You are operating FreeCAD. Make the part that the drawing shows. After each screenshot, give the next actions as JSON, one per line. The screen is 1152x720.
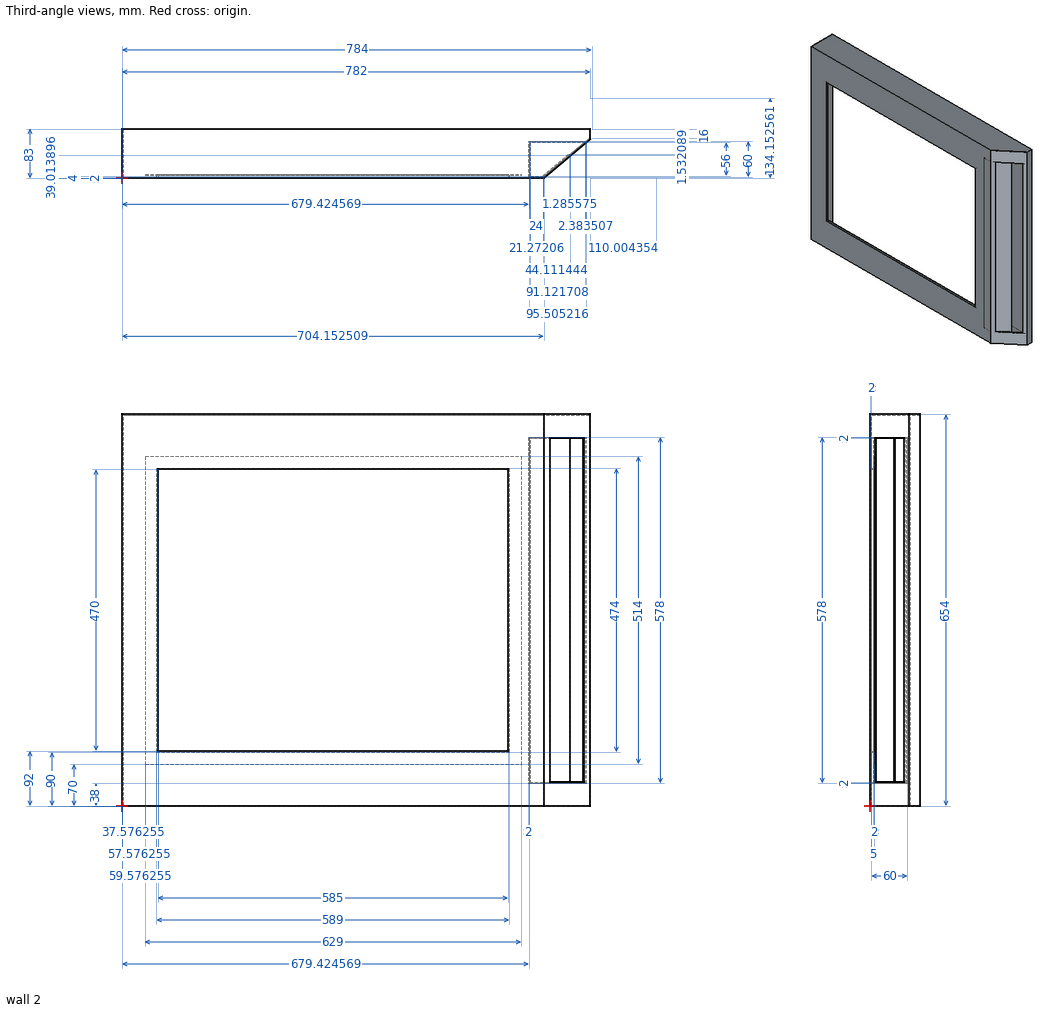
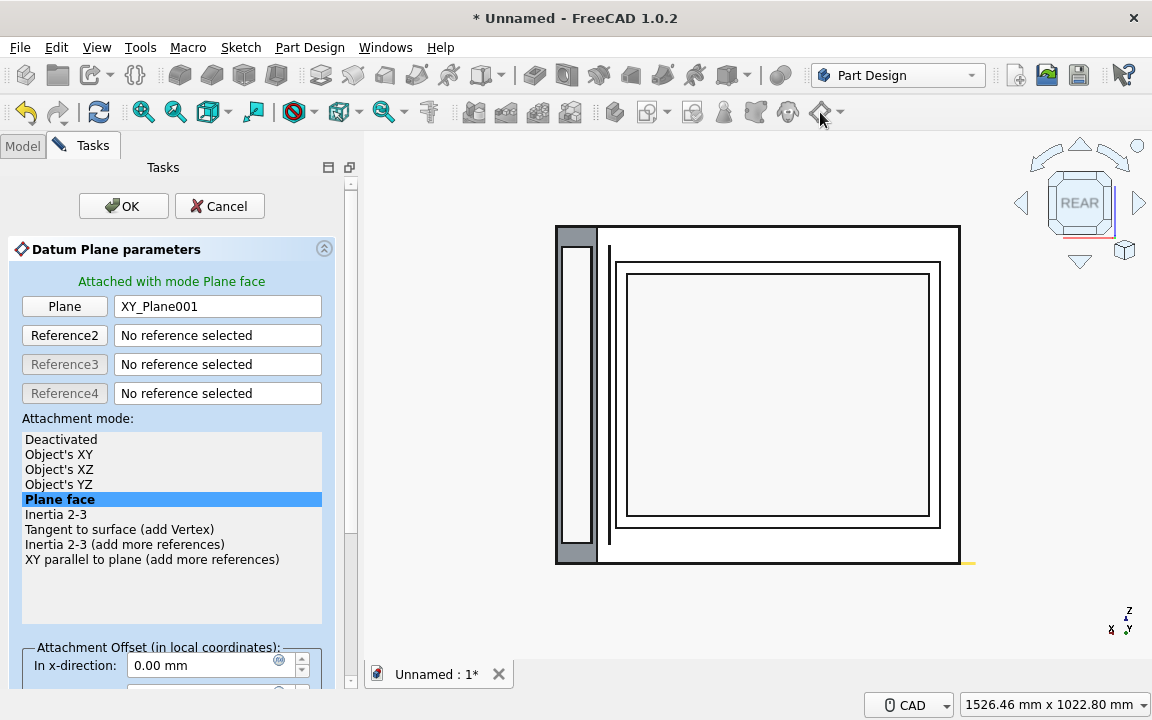
{"action": "scroll", "coordinate": [351, 432], "scroll_direction": "down", "scroll_amount": 2}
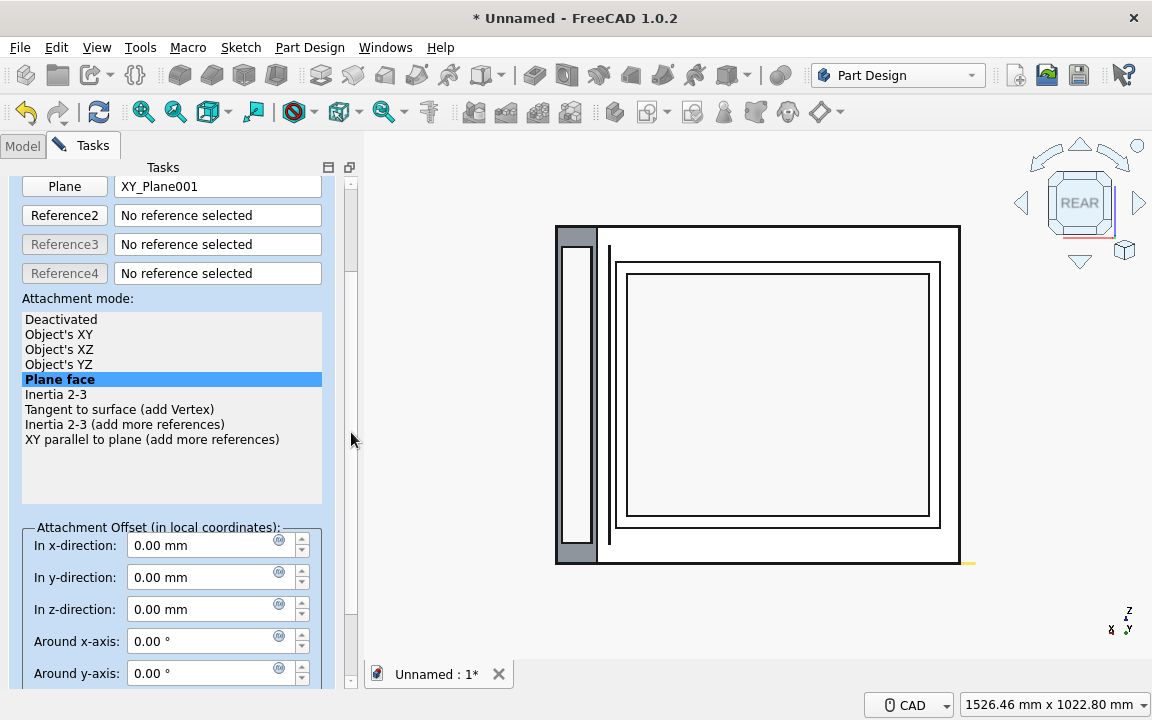
{"action": "triple_click", "coordinate": [210, 609]}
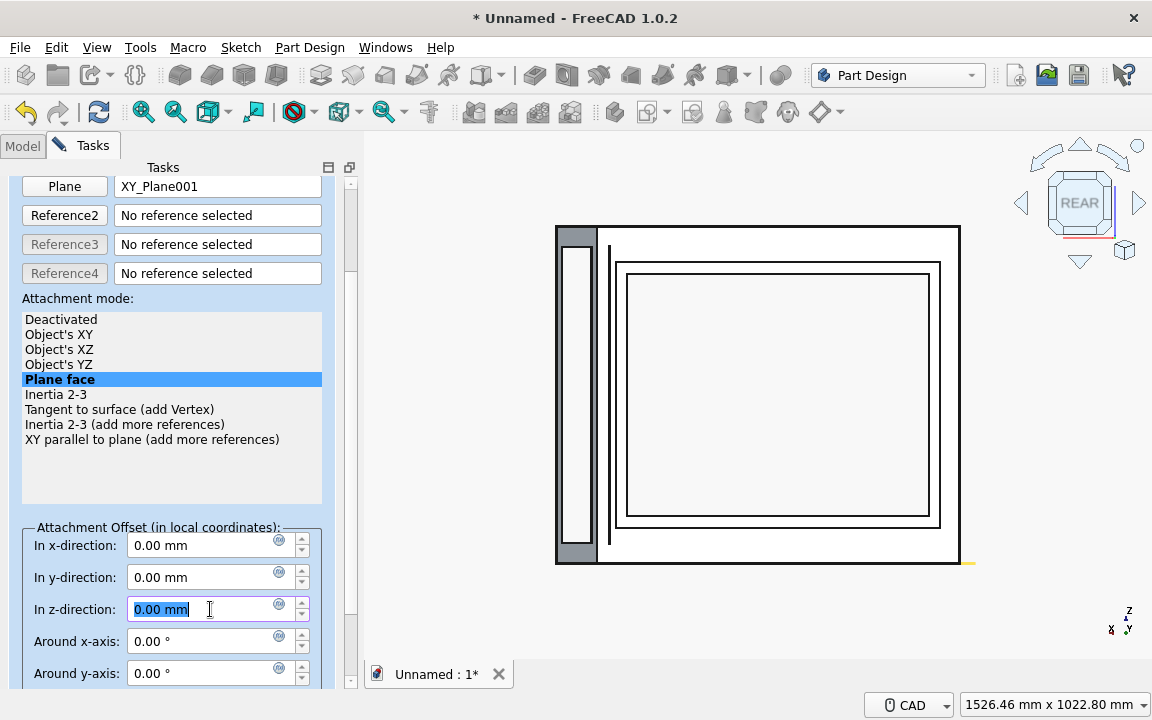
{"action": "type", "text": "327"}
{"action": "key", "text": "Tab"}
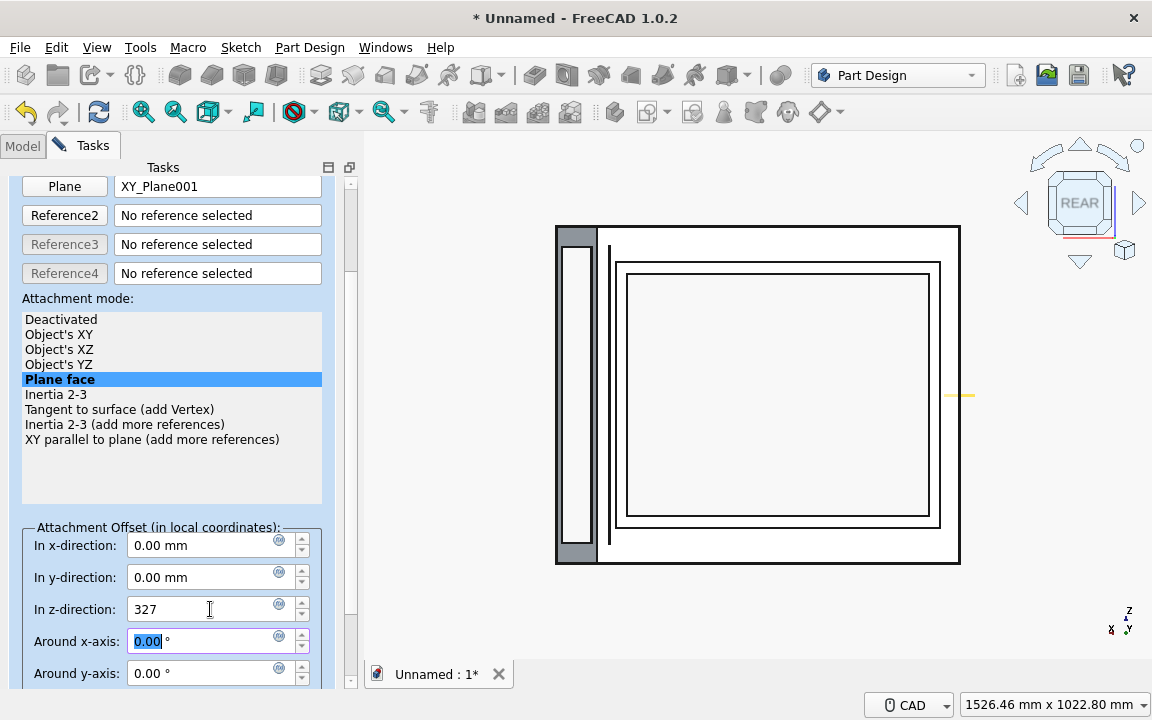
{"action": "scroll", "coordinate": [351, 432], "scroll_direction": "up", "scroll_amount": 3}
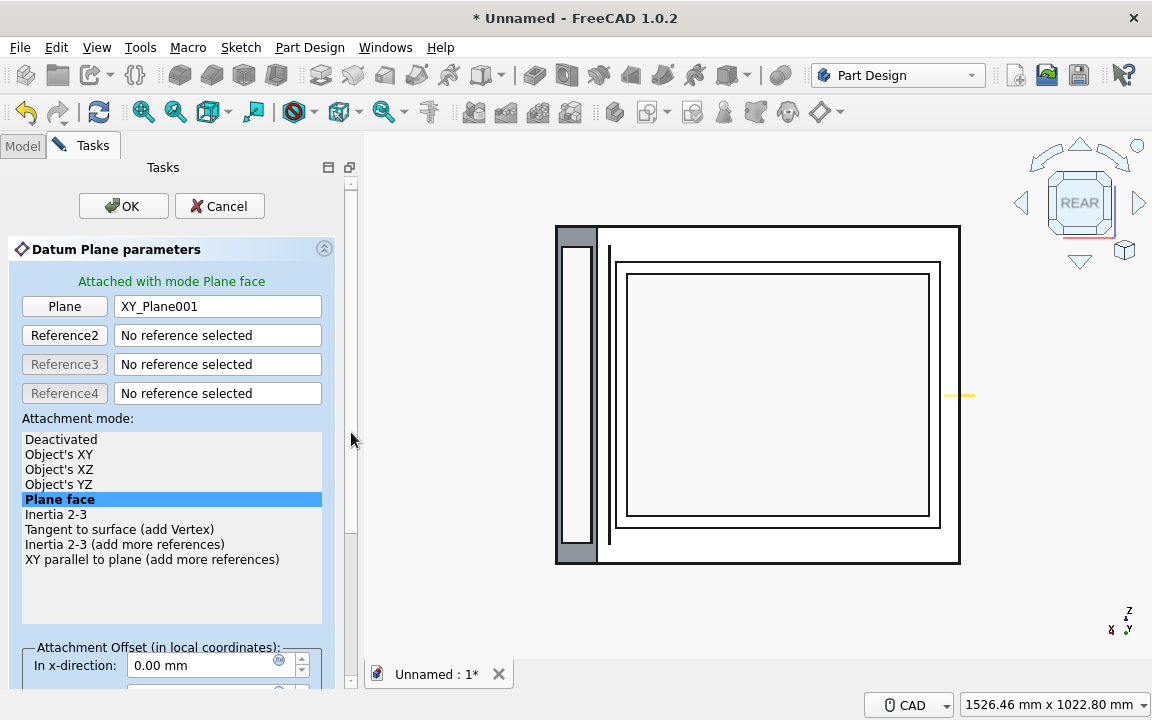
{"action": "left_click", "coordinate": [124, 206]}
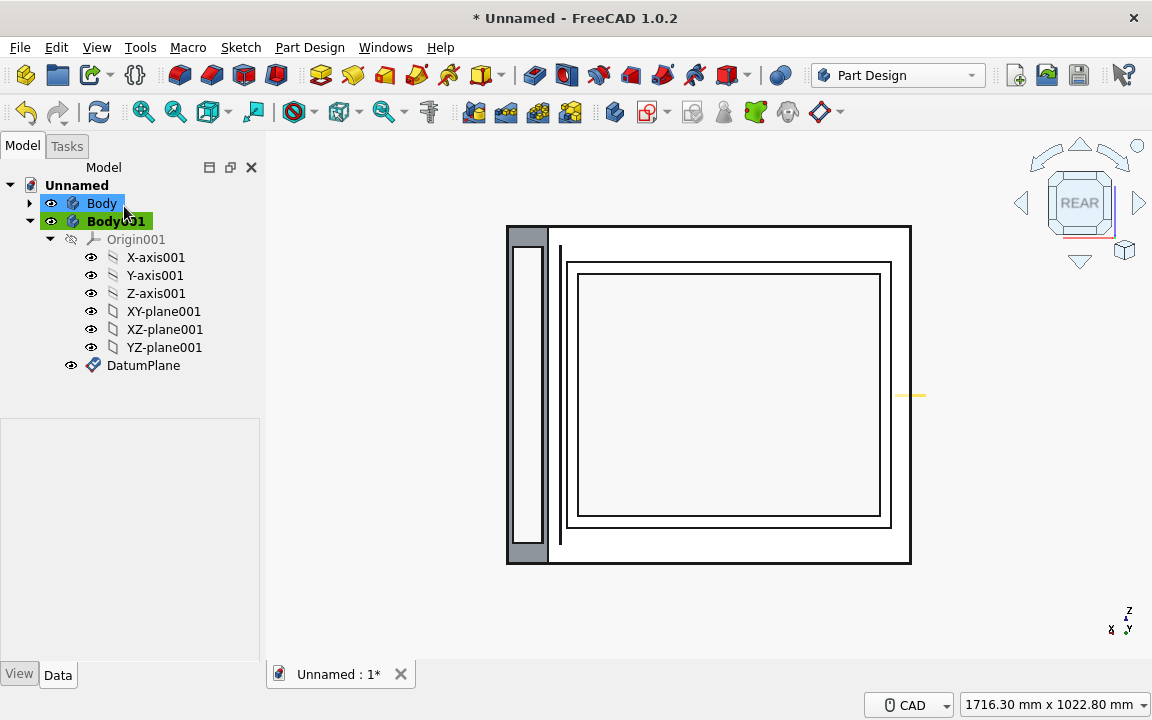
{"action": "left_click", "coordinate": [116, 365]}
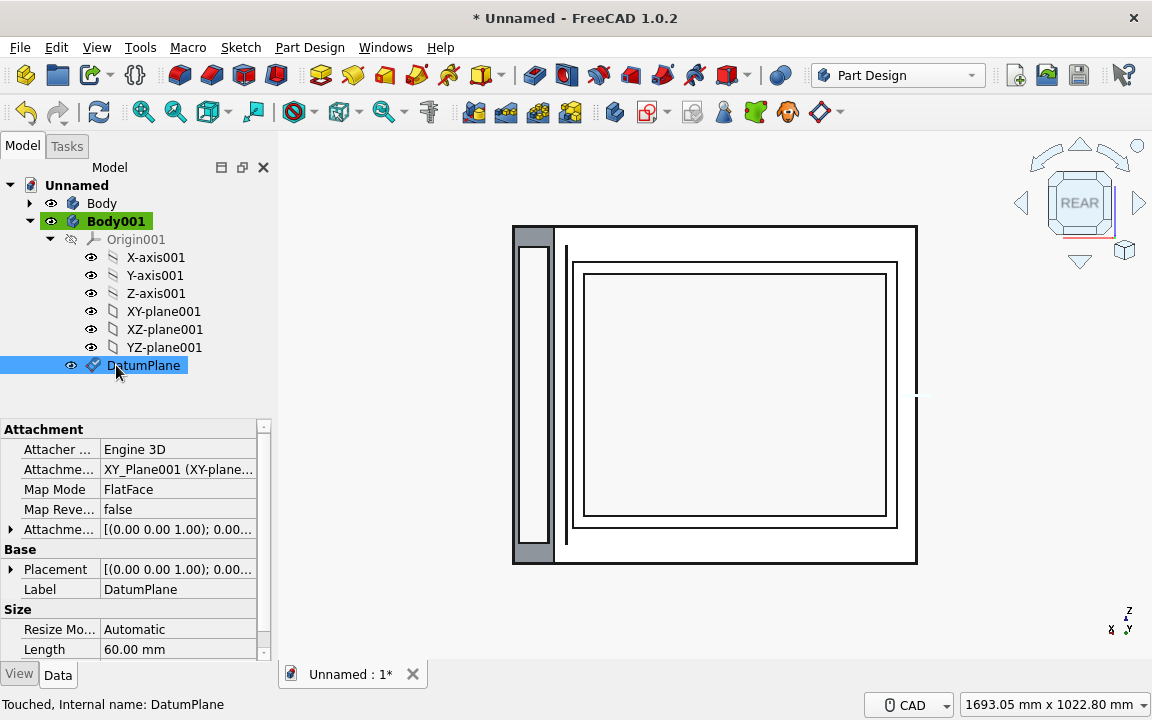
{"action": "left_click", "coordinate": [648, 112]}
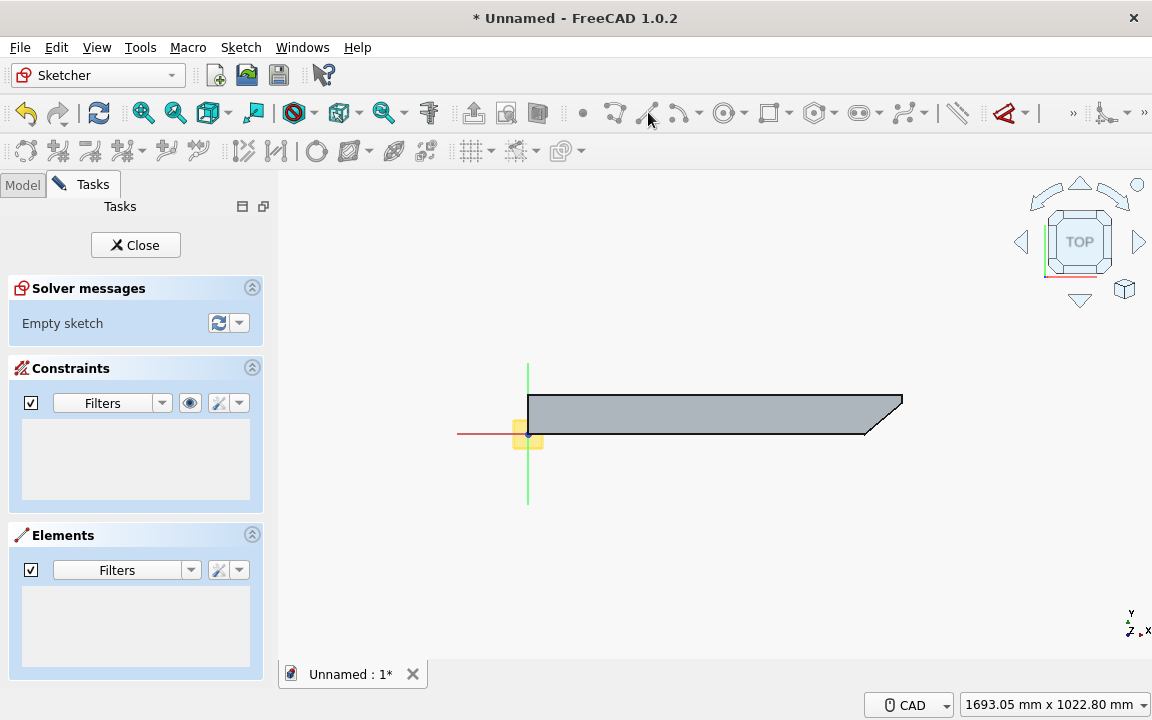
{"action": "scroll", "coordinate": [893, 419], "scroll_direction": "up", "scroll_amount": 12}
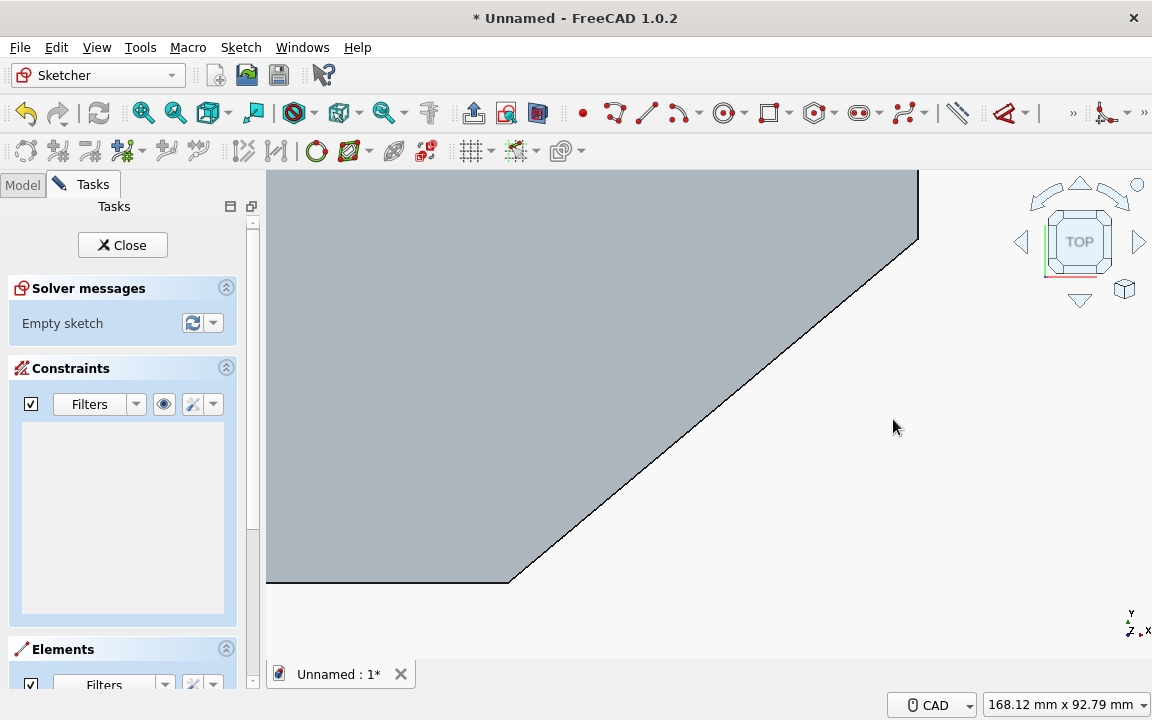
{"action": "key", "text": "g m"}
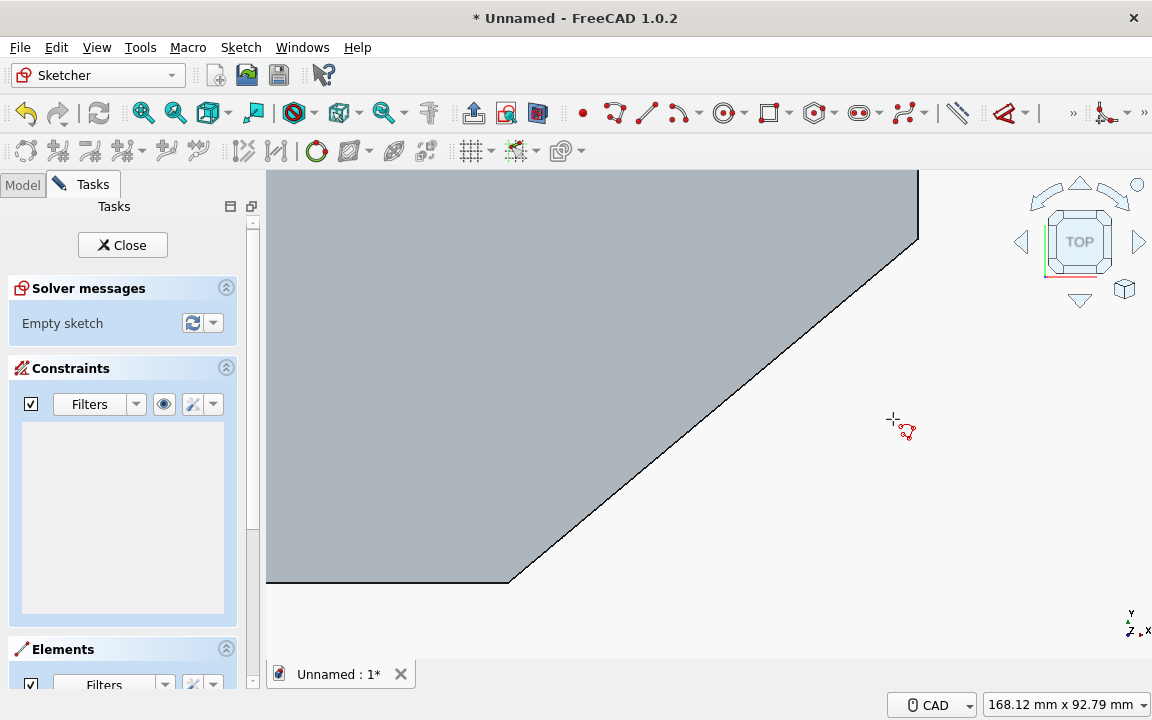
{"action": "scroll", "coordinate": [378, 572], "scroll_direction": "up", "scroll_amount": 3}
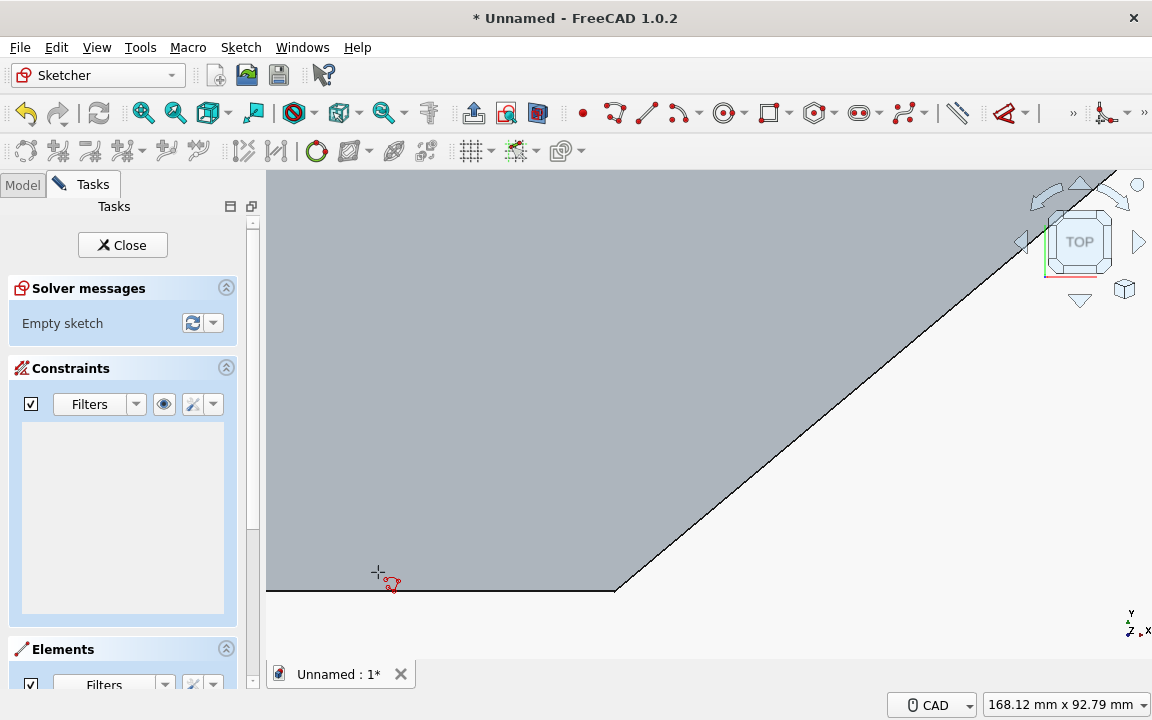
{"action": "left_click", "coordinate": [377, 572]}
{"action": "left_click", "coordinate": [608, 572]}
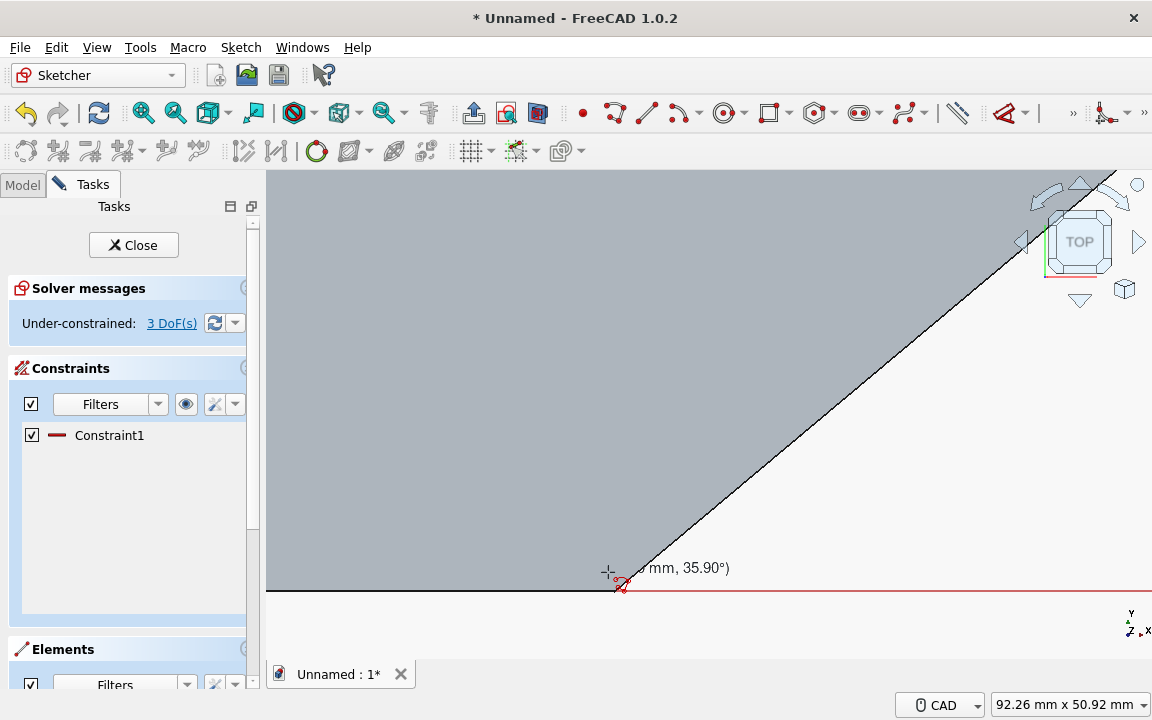
{"action": "scroll", "coordinate": [403, 573], "scroll_direction": "down", "scroll_amount": 3}